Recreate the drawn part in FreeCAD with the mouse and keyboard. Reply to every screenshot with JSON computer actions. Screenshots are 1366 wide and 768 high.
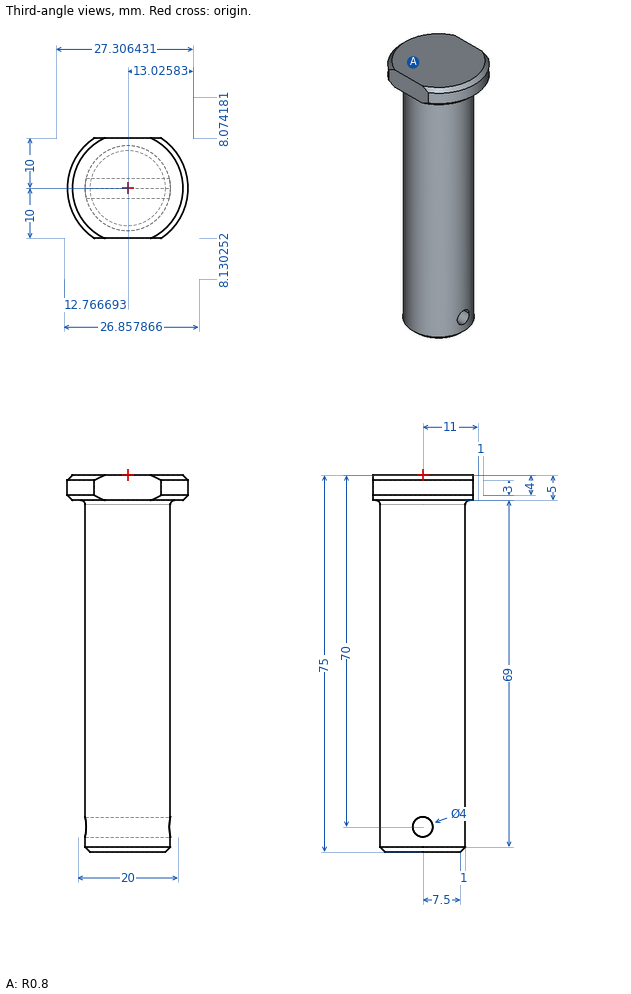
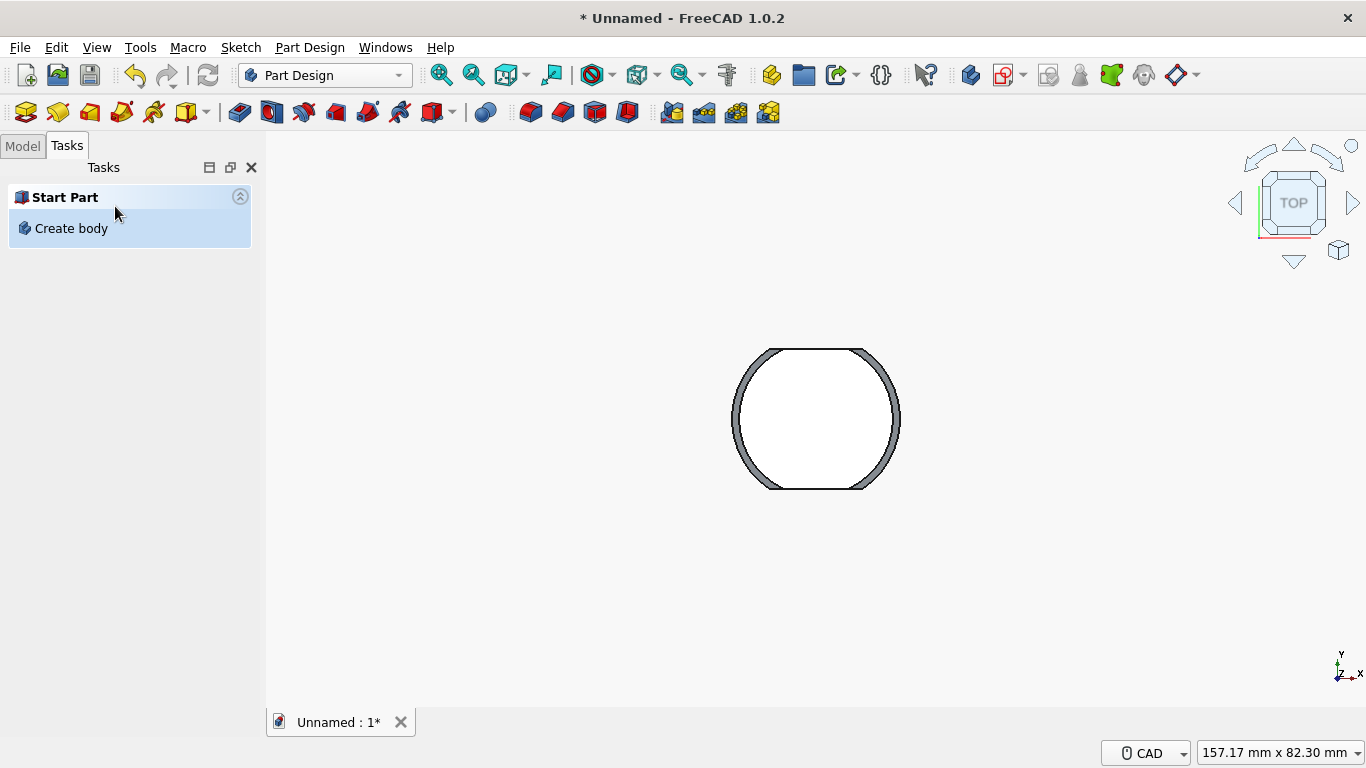
{"action": "left_click", "coordinate": [442, 76]}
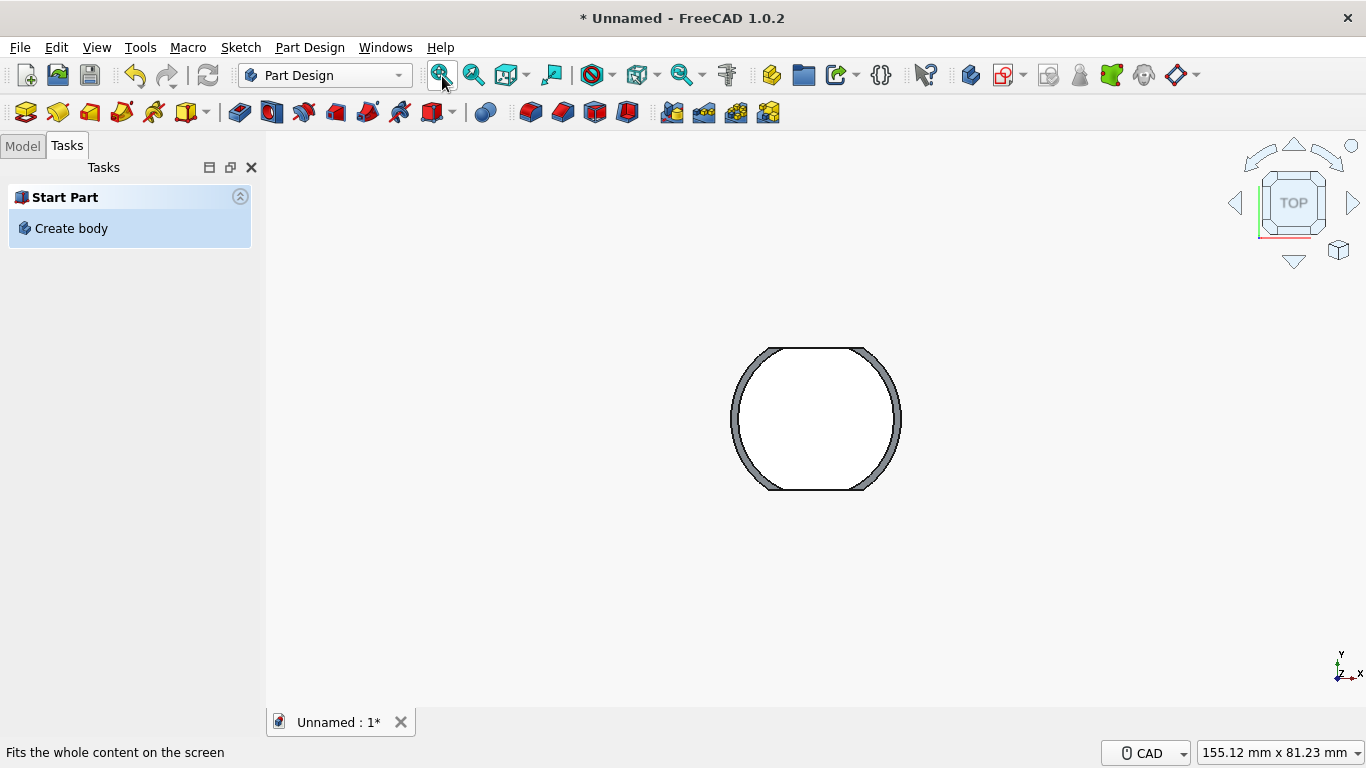
{"action": "key", "text": "1"}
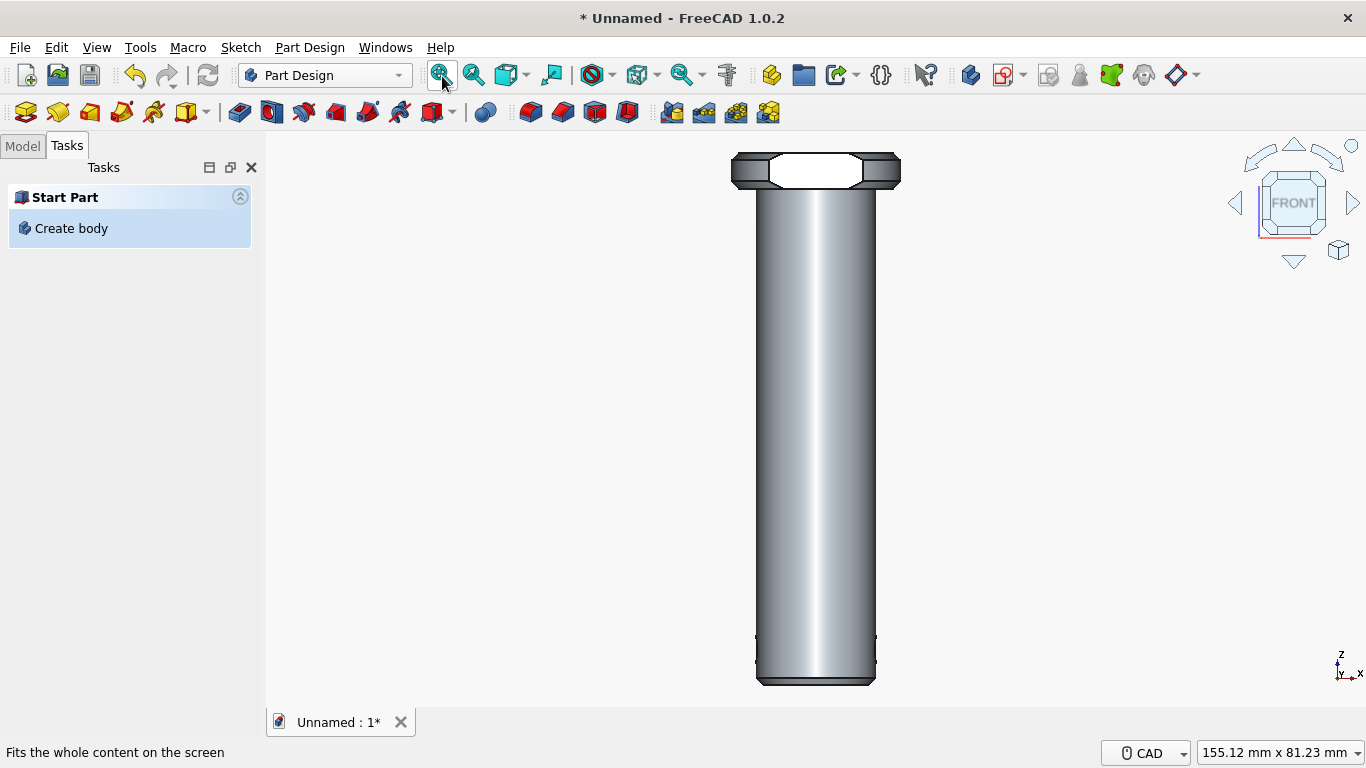
{"action": "key", "text": "3"}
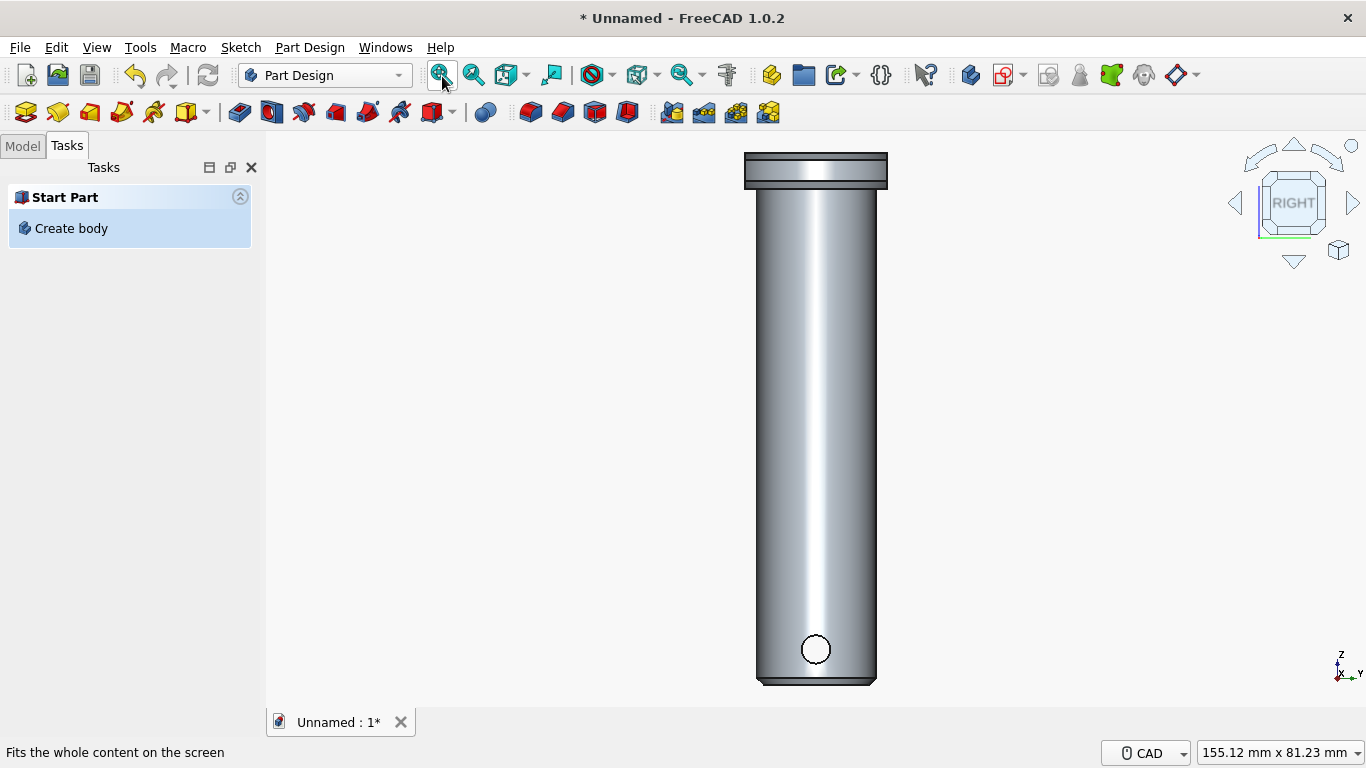
{"action": "key", "text": "5"}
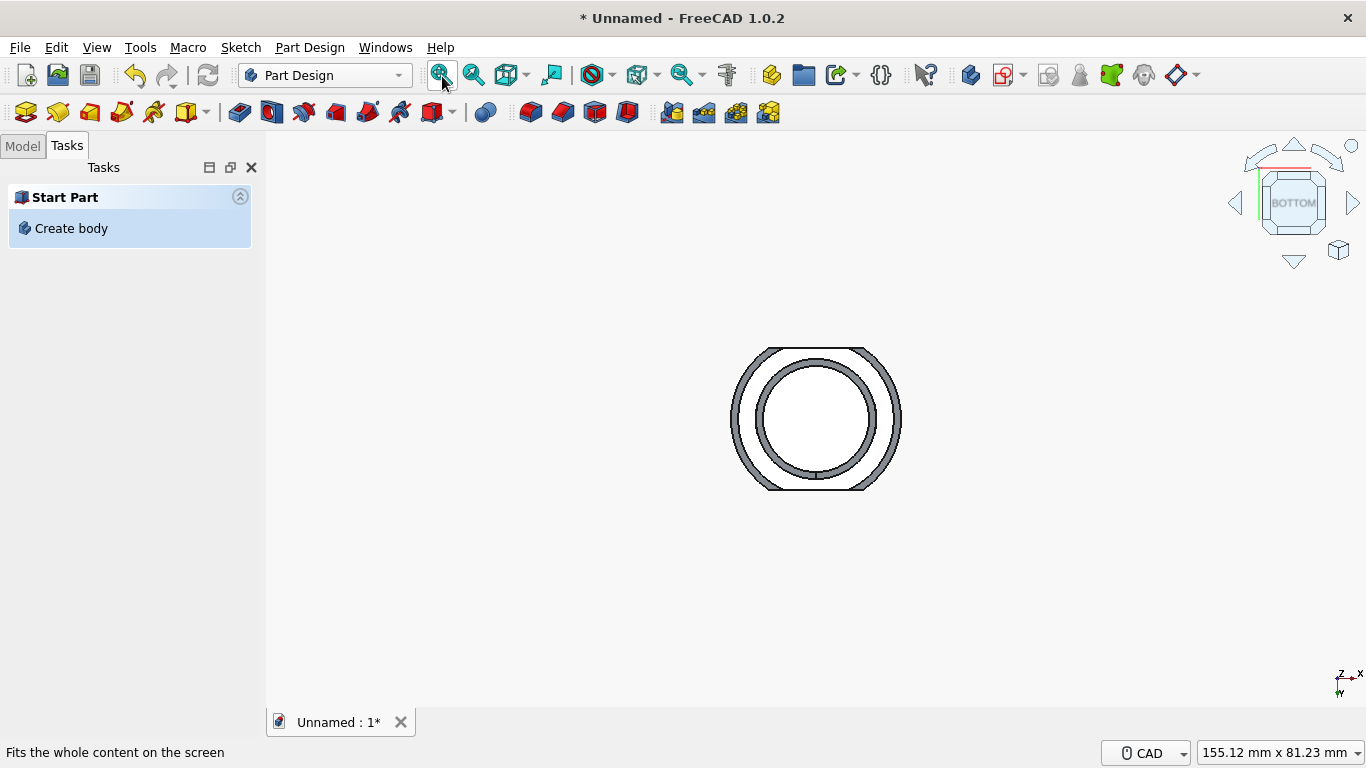
{"action": "left_click", "coordinate": [442, 76]}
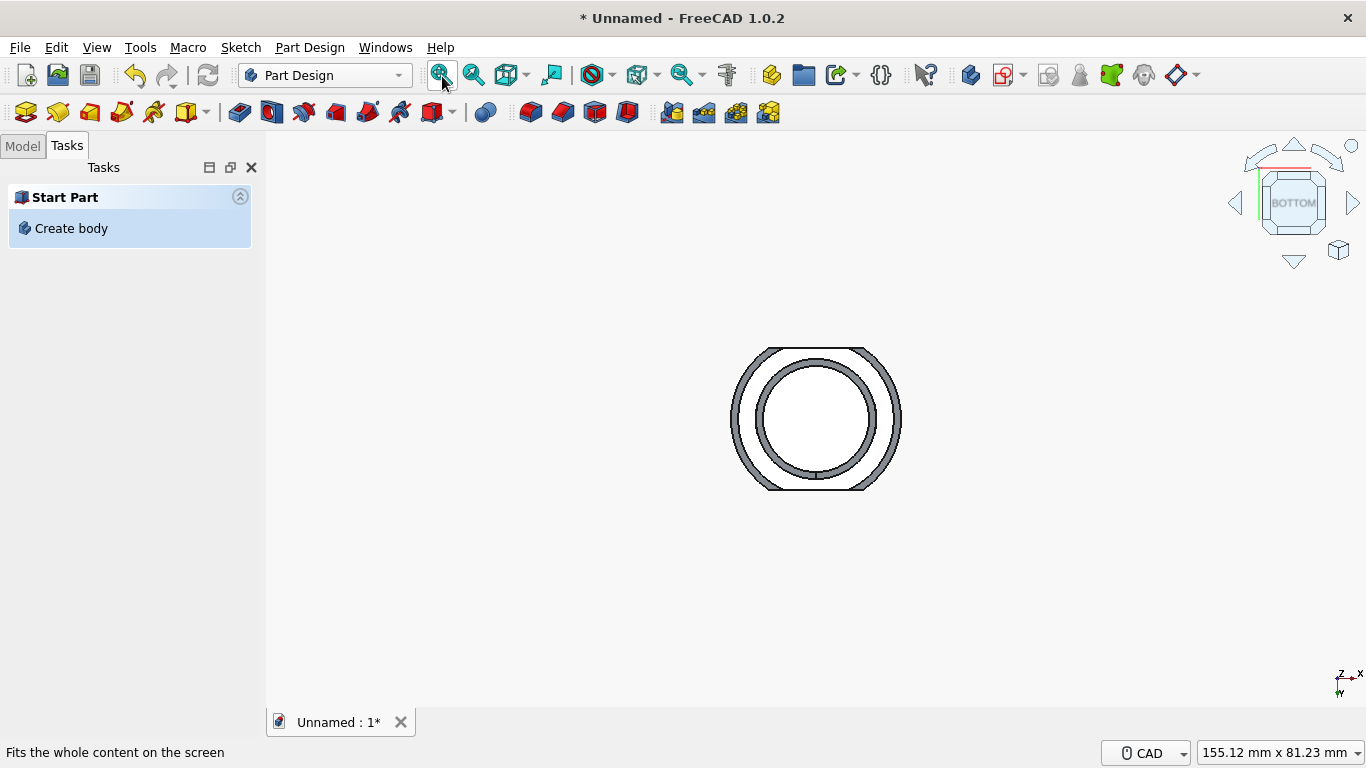
{"action": "key", "text": "4"}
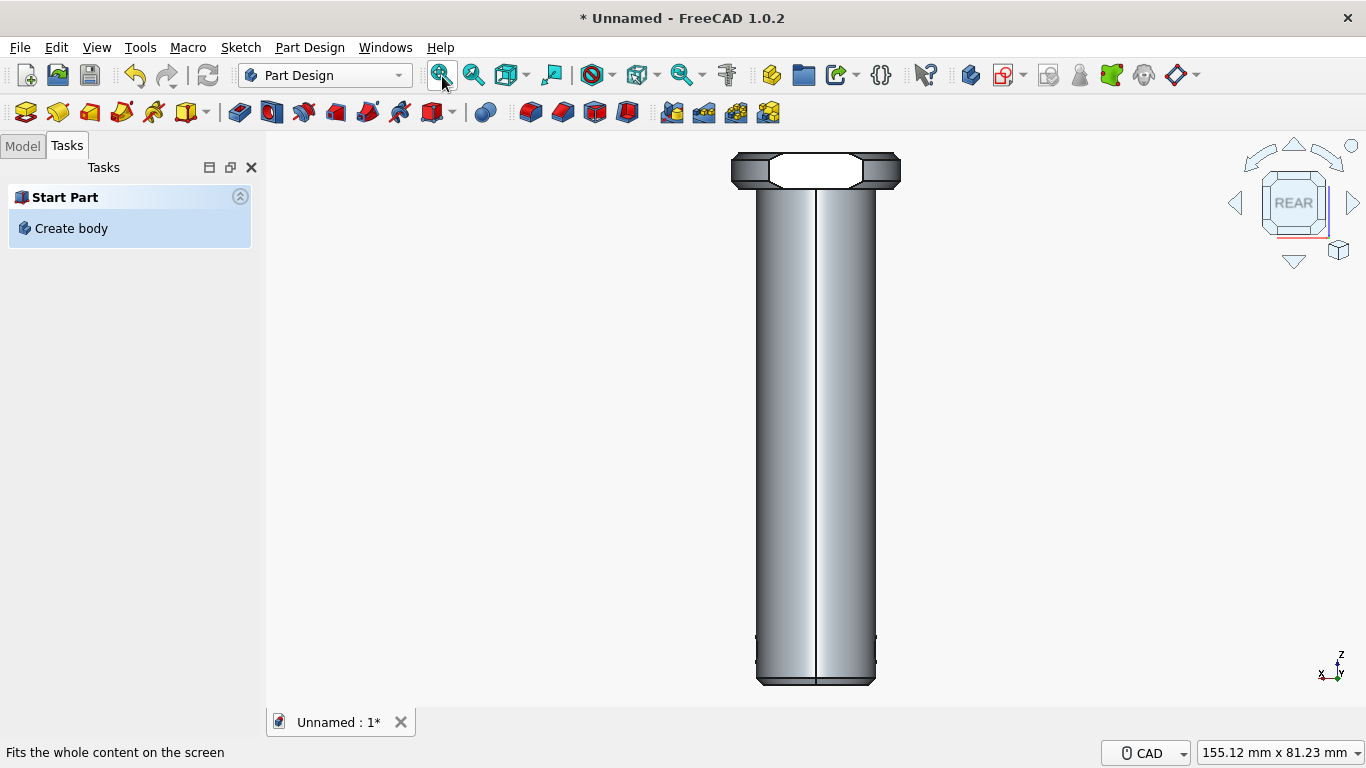
{"action": "key", "text": "6"}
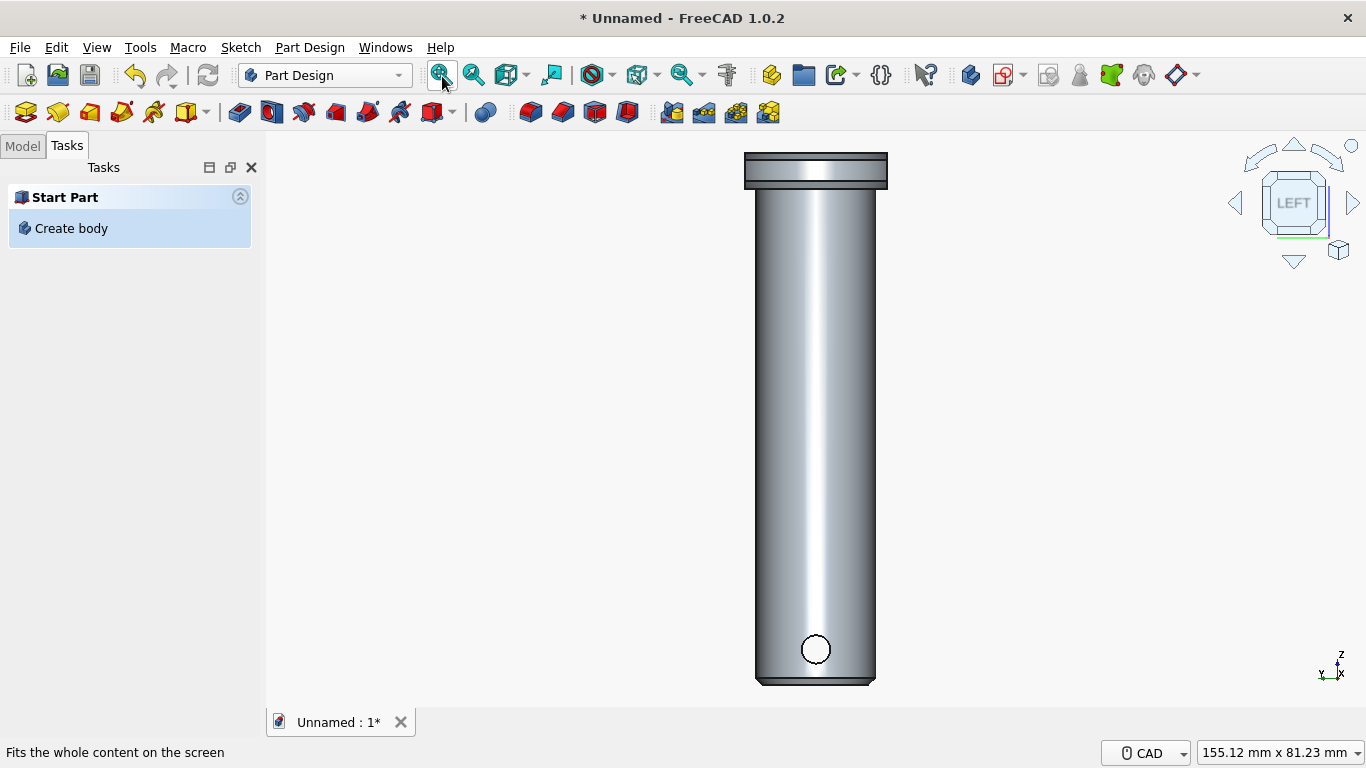
{"action": "key", "text": "v 3"}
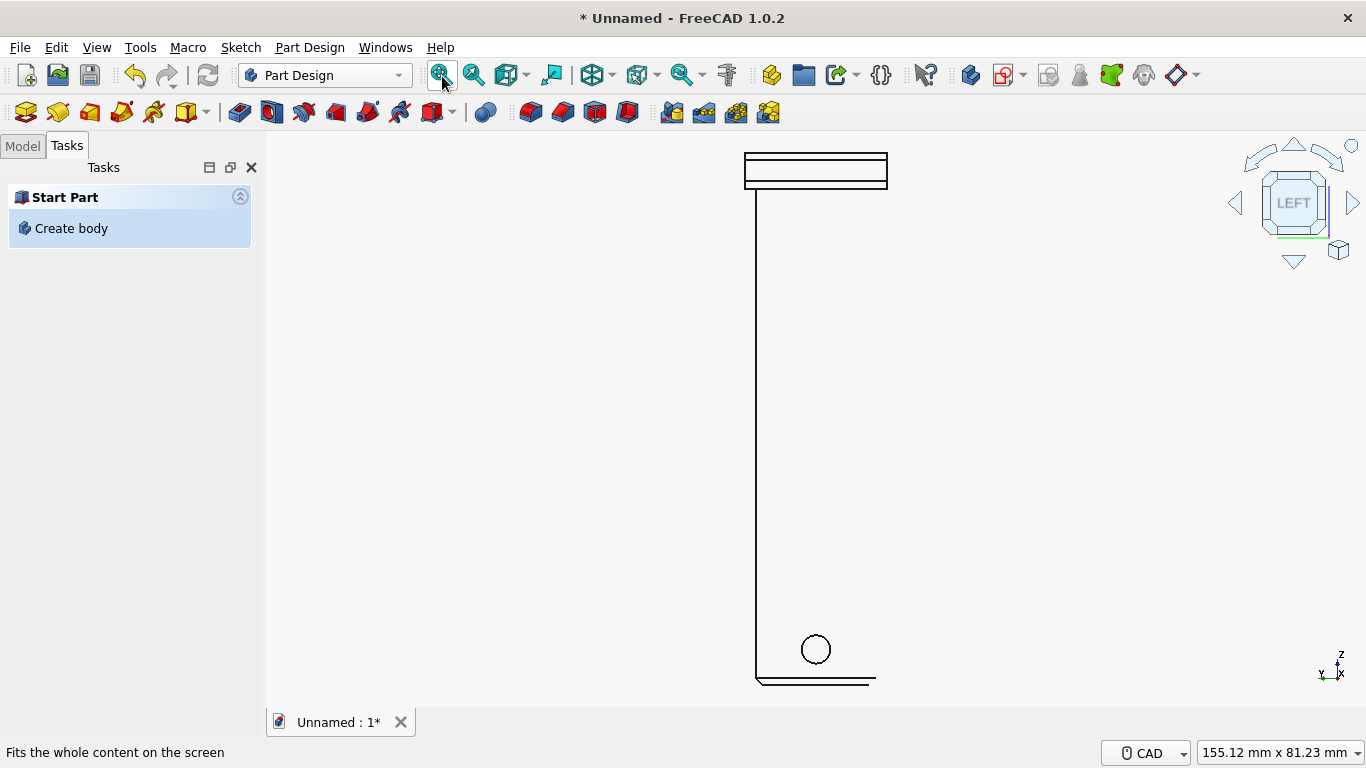
{"action": "key", "text": "0"}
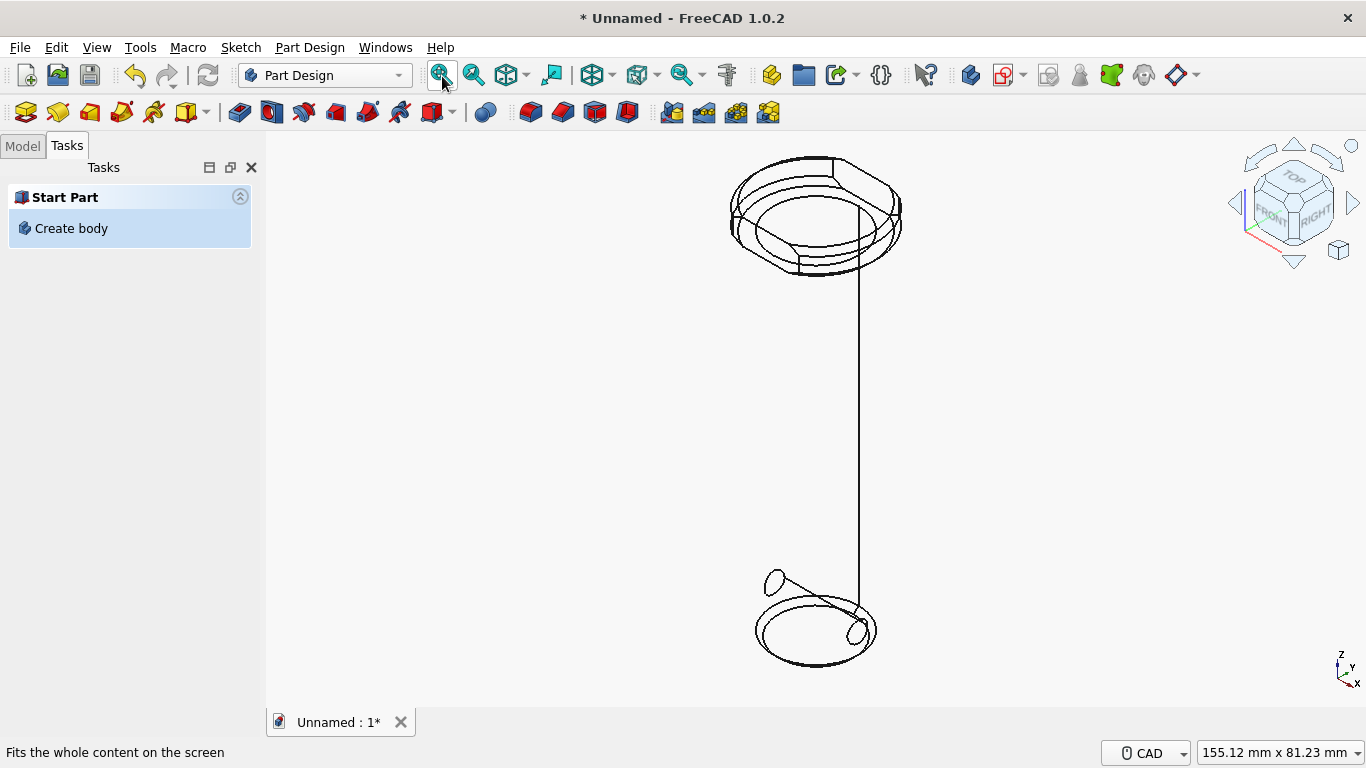
{"action": "left_click", "coordinate": [773, 254]}